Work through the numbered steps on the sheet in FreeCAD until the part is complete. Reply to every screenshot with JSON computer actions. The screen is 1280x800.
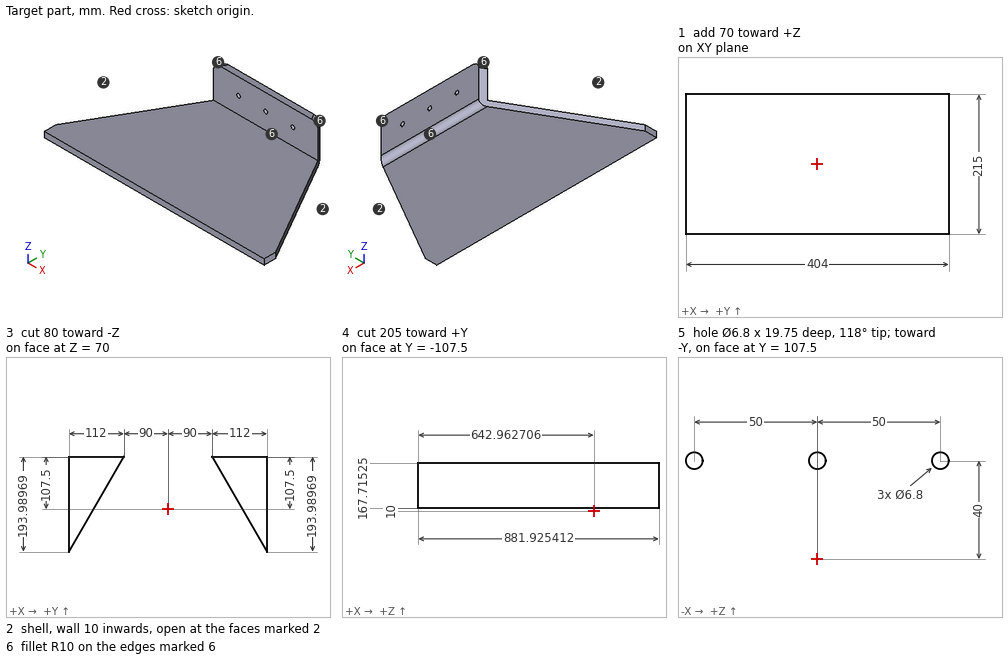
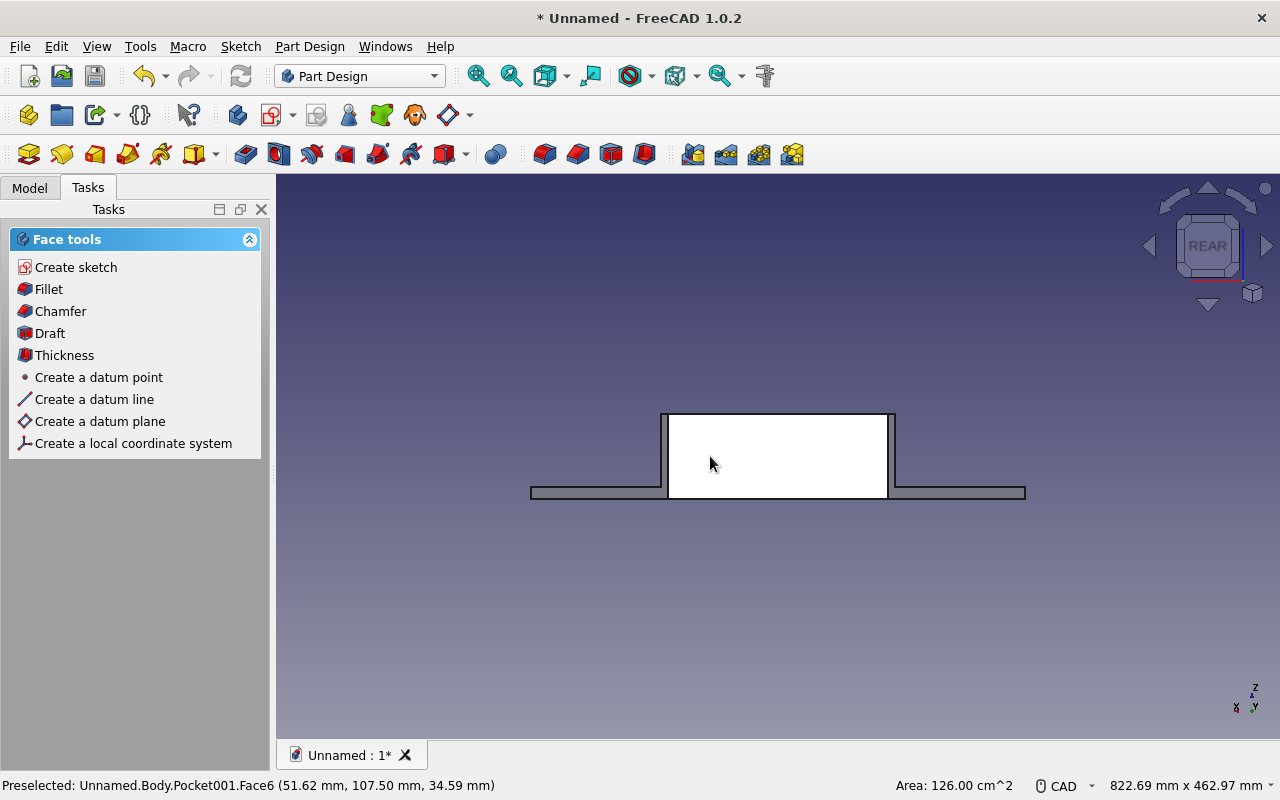
{"action": "left_click", "coordinate": [270, 116]}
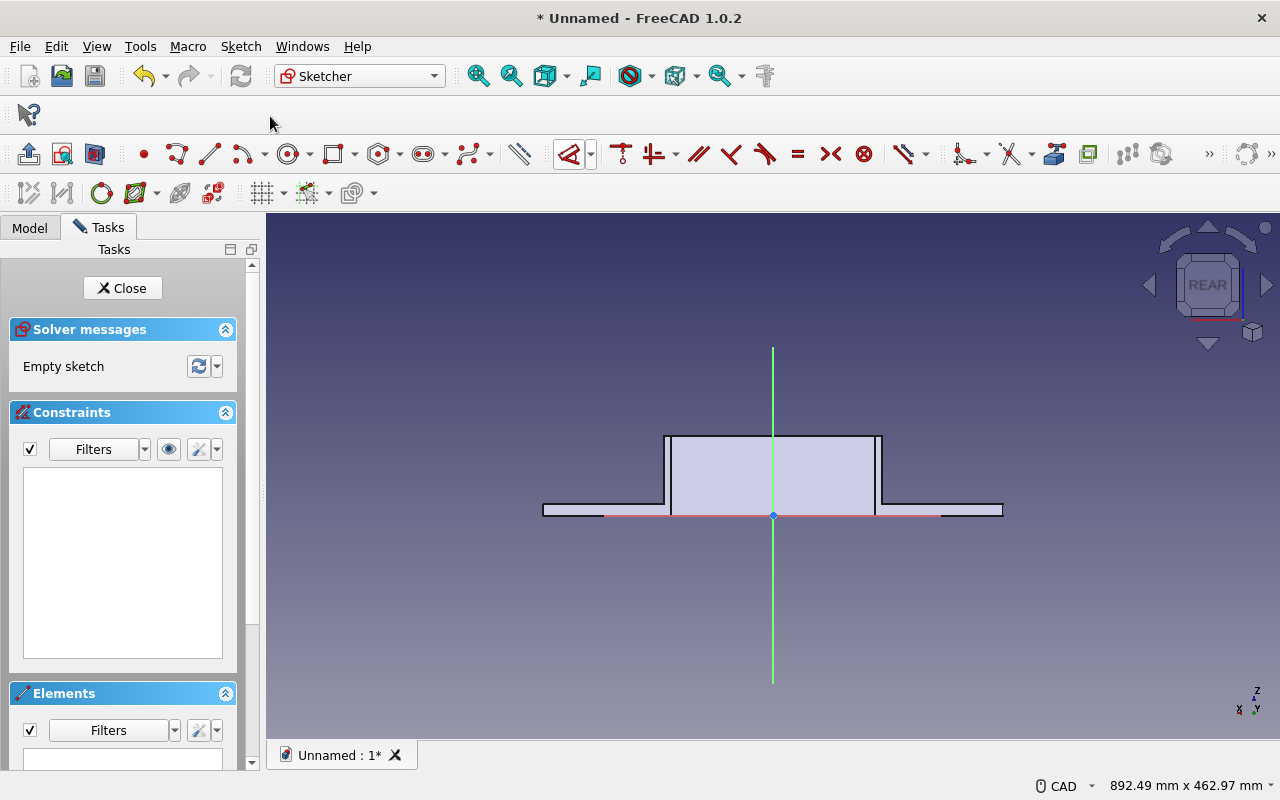
{"action": "scroll", "coordinate": [790, 495], "scroll_direction": "up", "scroll_amount": 8}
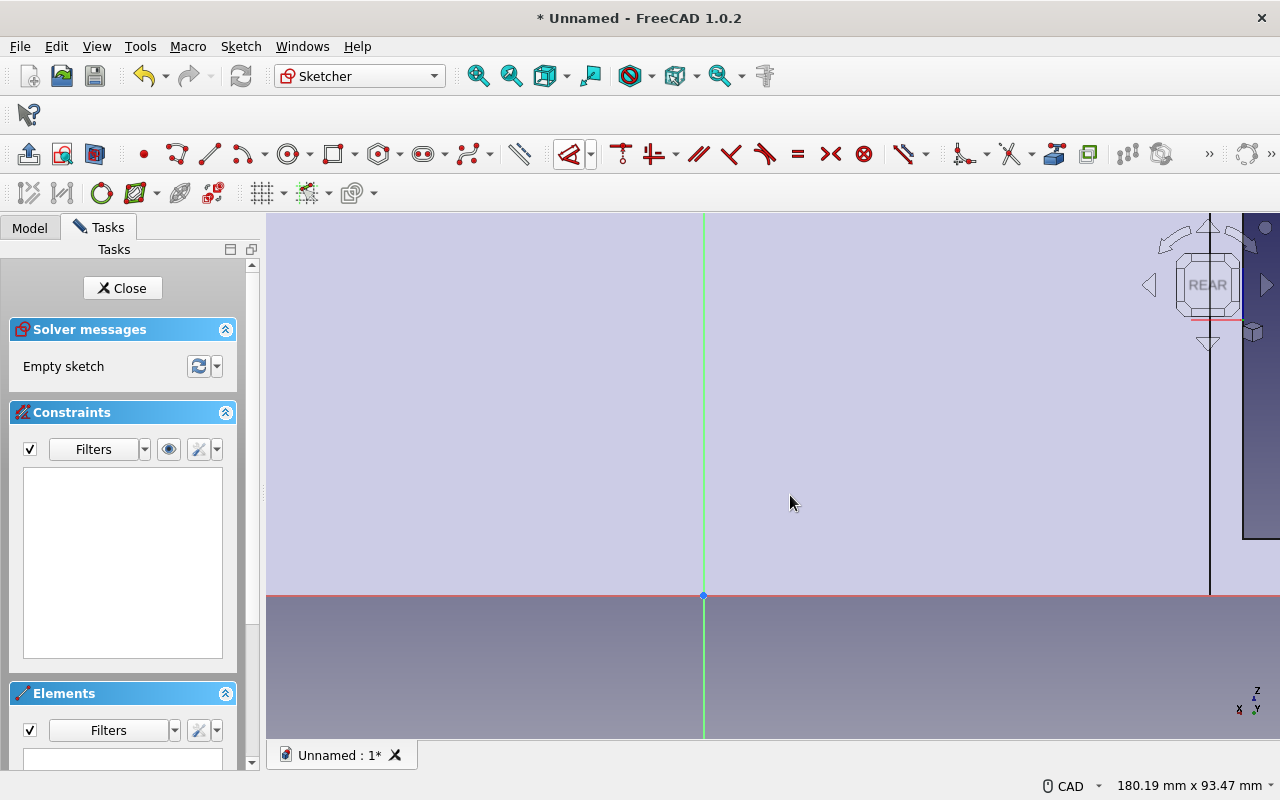
{"action": "left_click", "coordinate": [288, 154]}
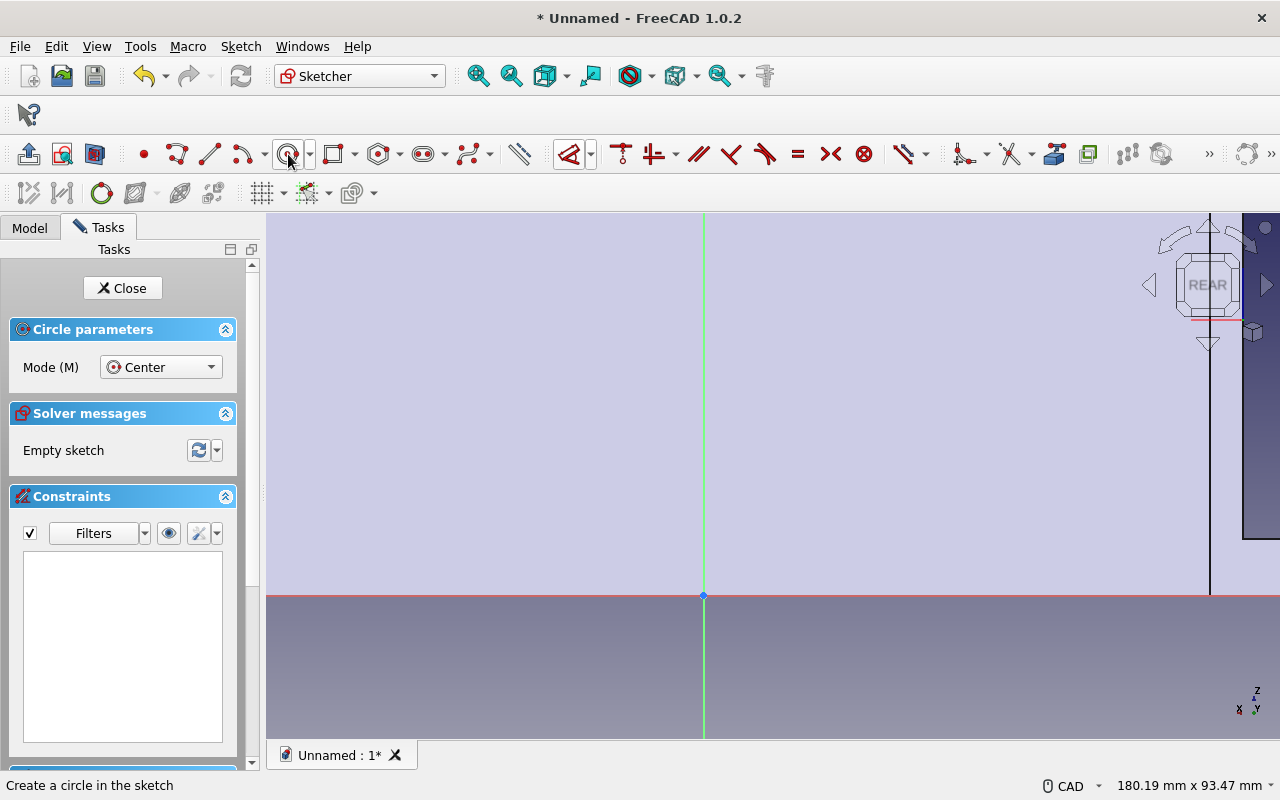
{"action": "left_click", "coordinate": [985, 371]}
{"action": "left_click", "coordinate": [999, 357]}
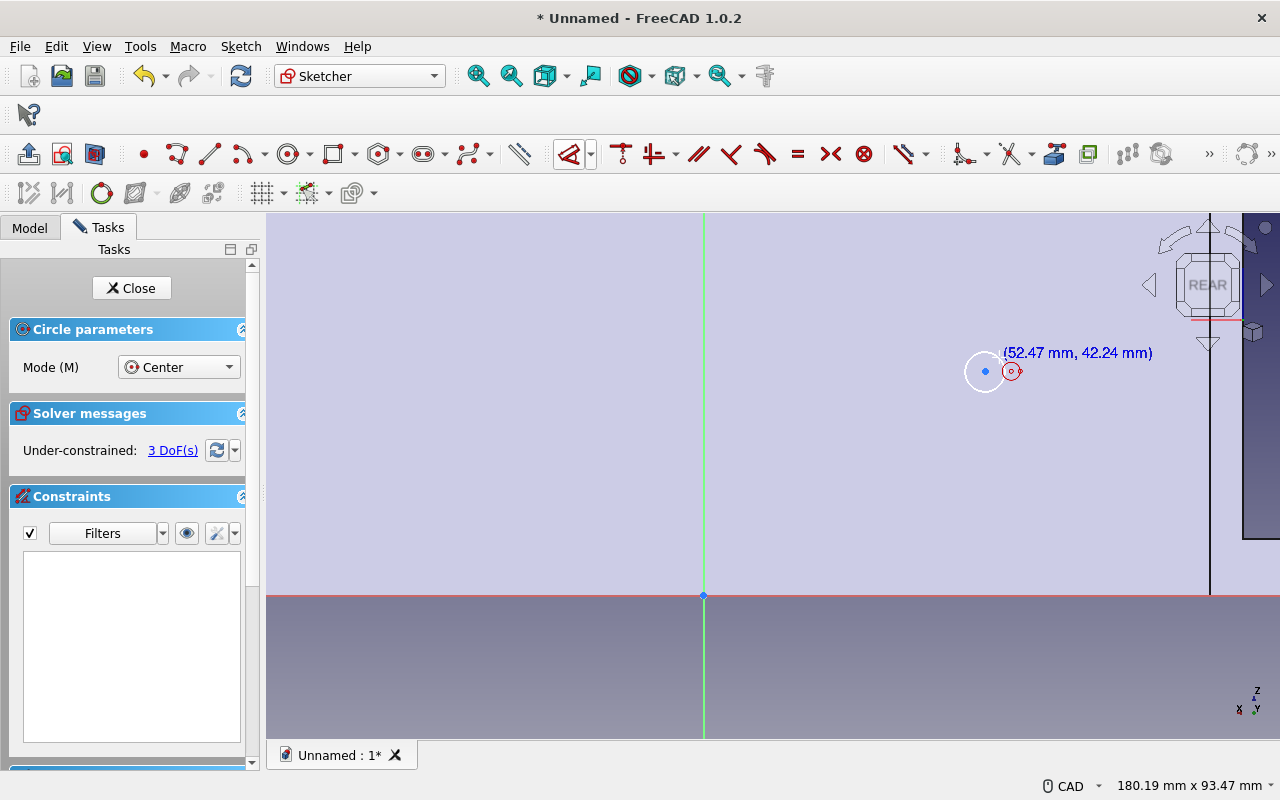
{"action": "left_click", "coordinate": [704, 371]}
{"action": "left_click", "coordinate": [722, 364]}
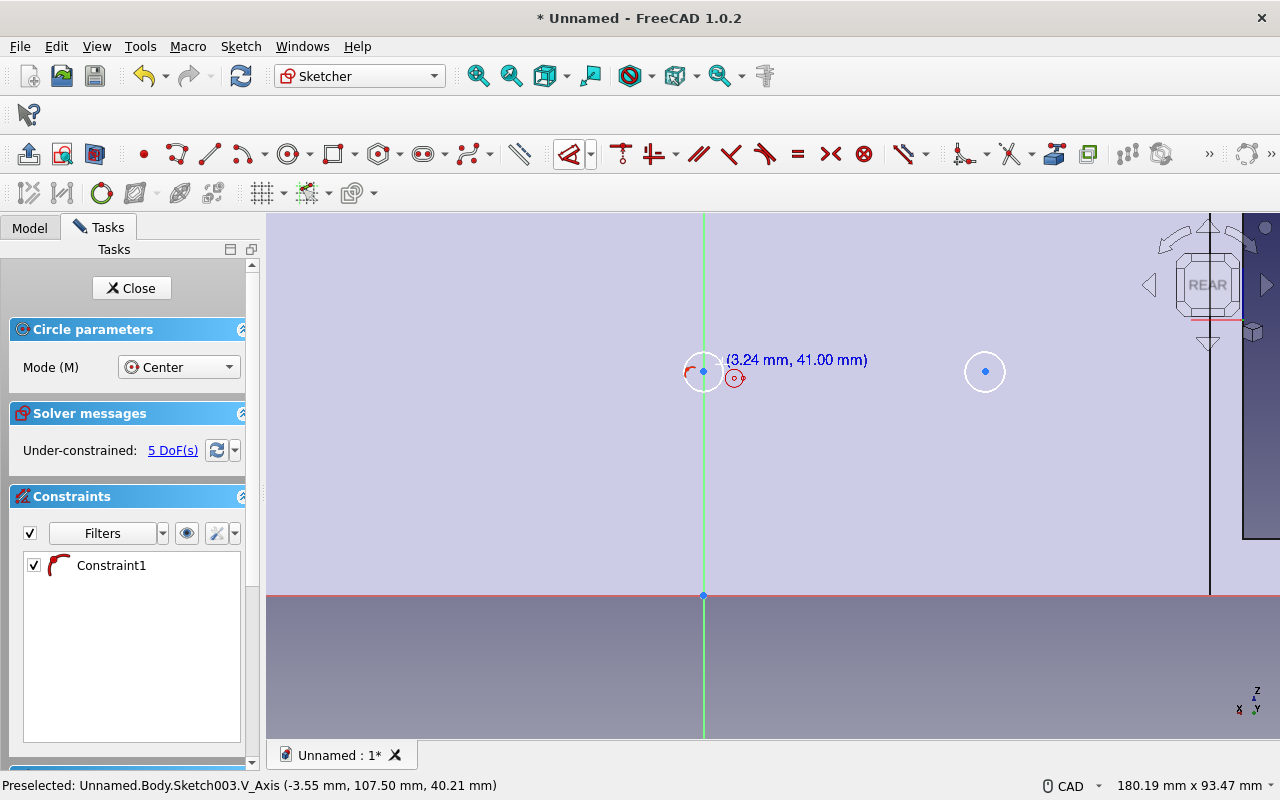
{"action": "left_click", "coordinate": [422, 371]}
{"action": "left_click", "coordinate": [436, 357]}
{"action": "key", "text": "Escape"}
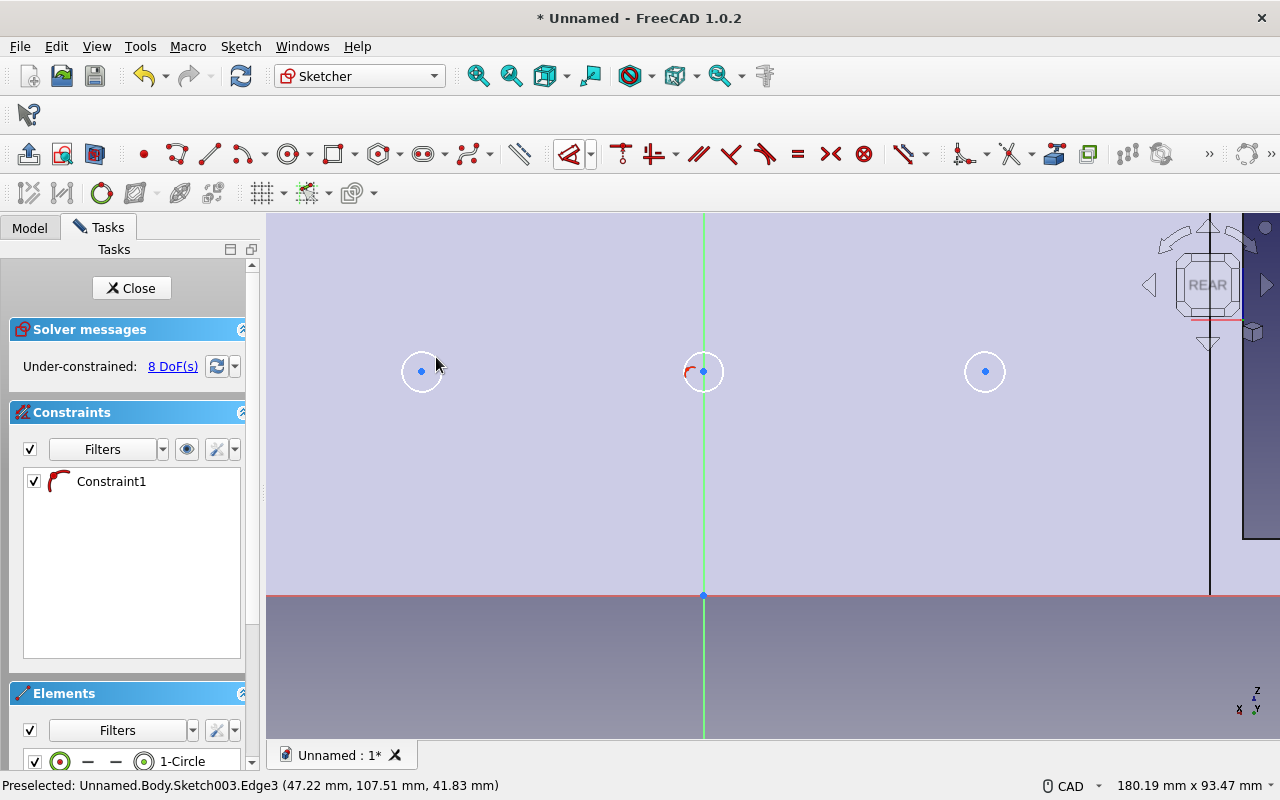
{"action": "left_click", "coordinate": [999, 358]}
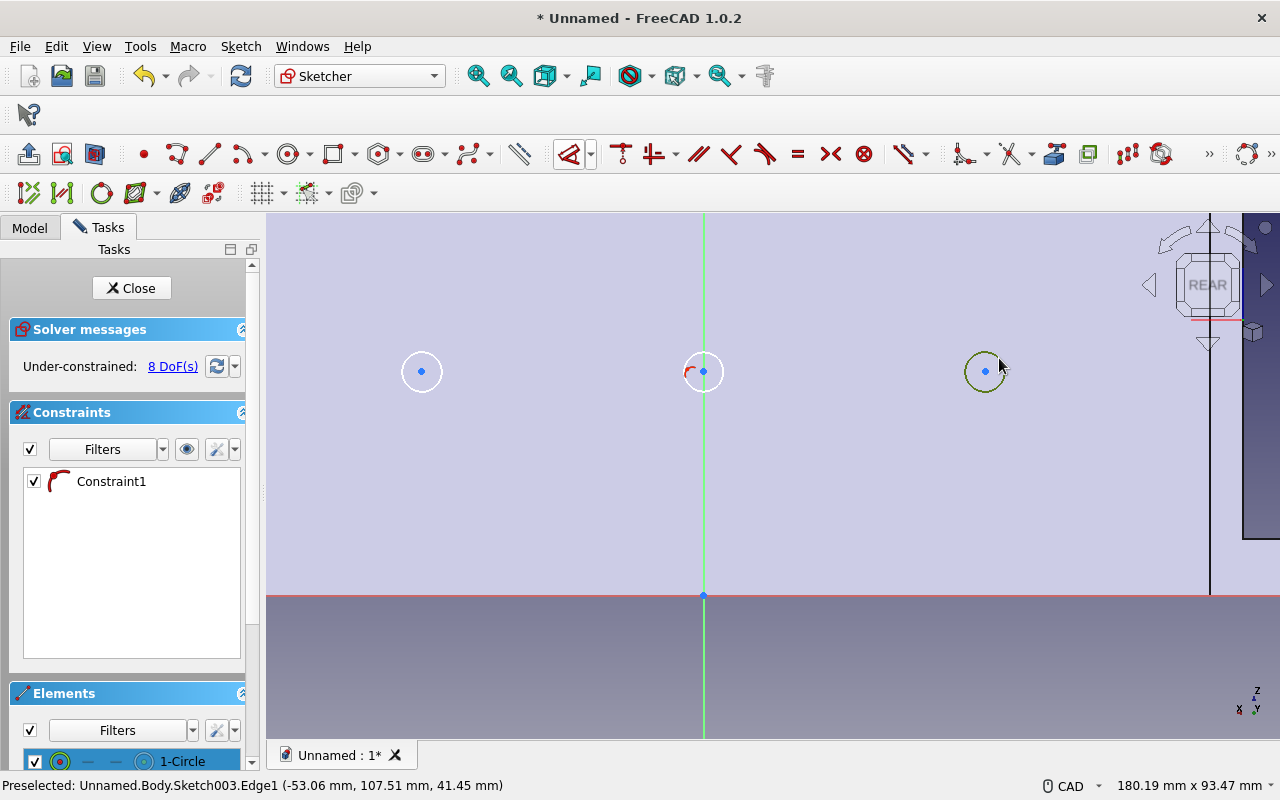
{"action": "left_click", "coordinate": [718, 358]}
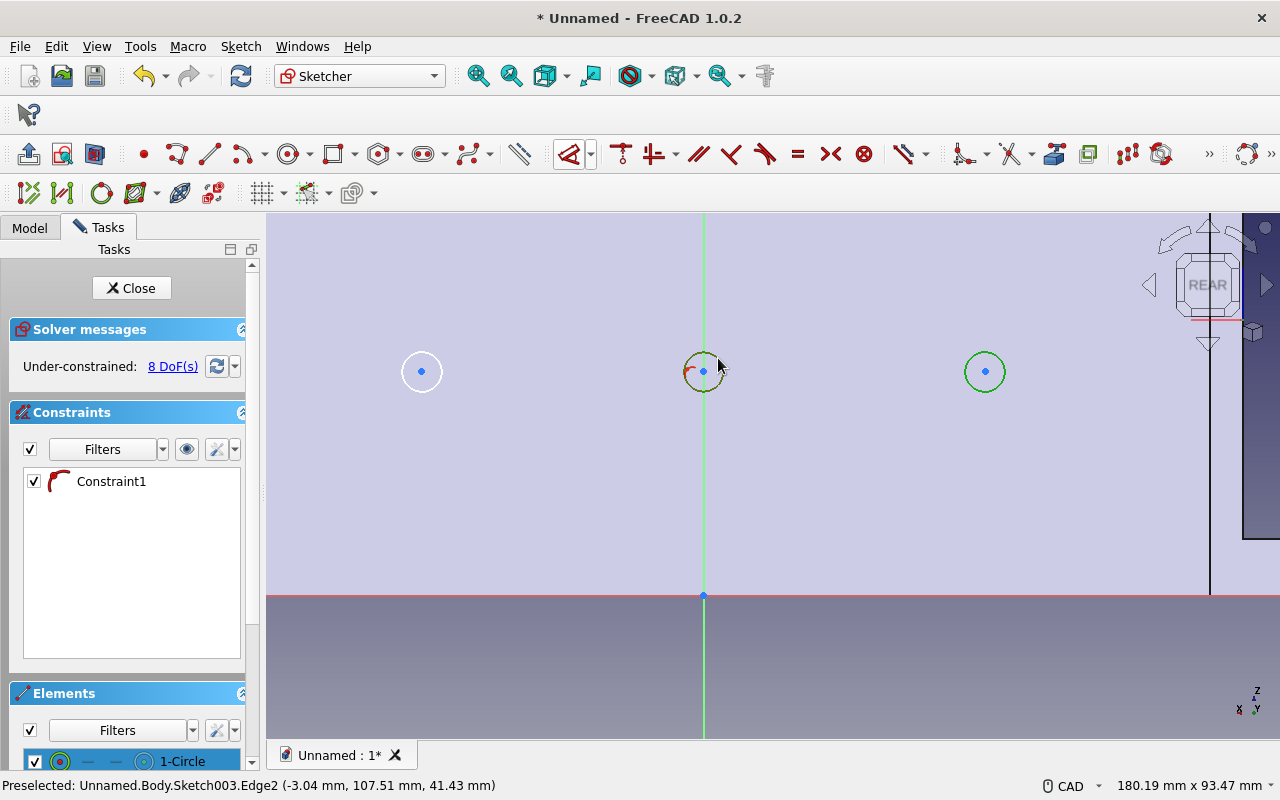
{"action": "left_click", "coordinate": [436, 358]}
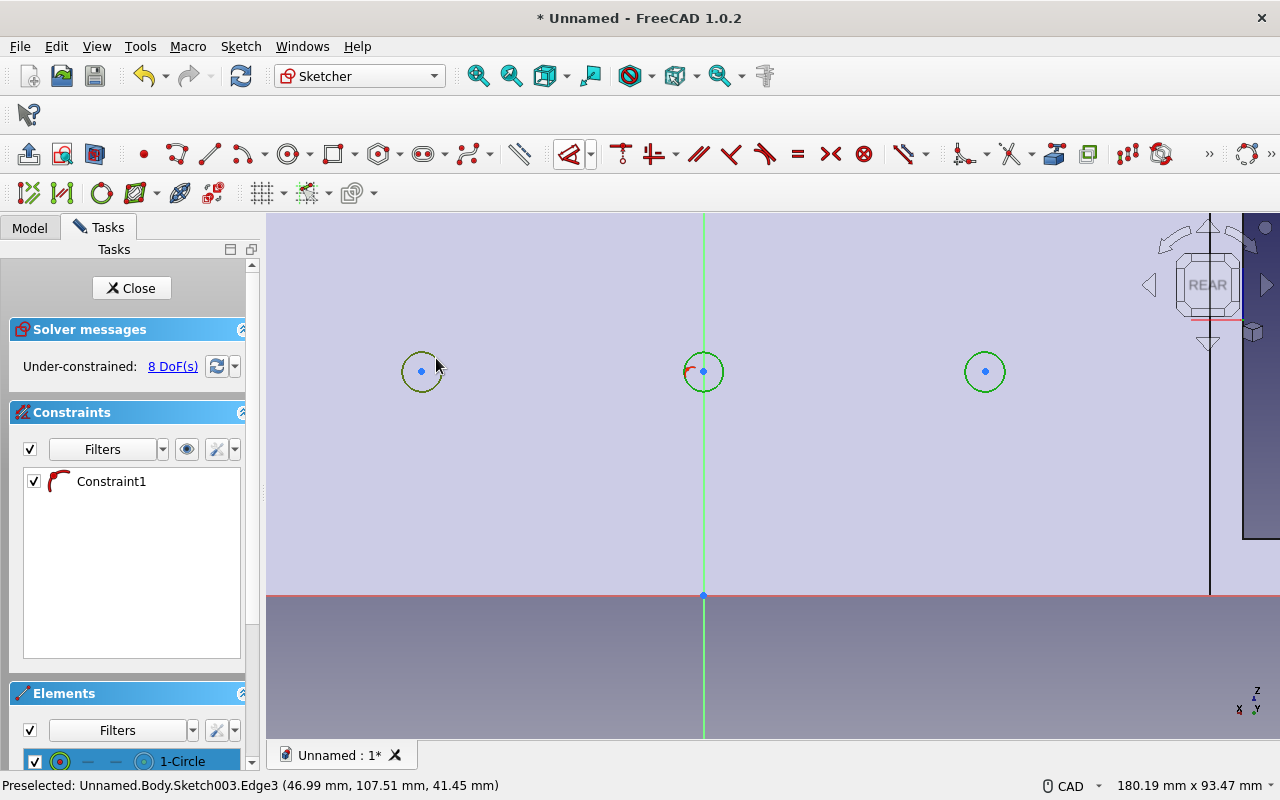
{"action": "left_click", "coordinate": [798, 154]}